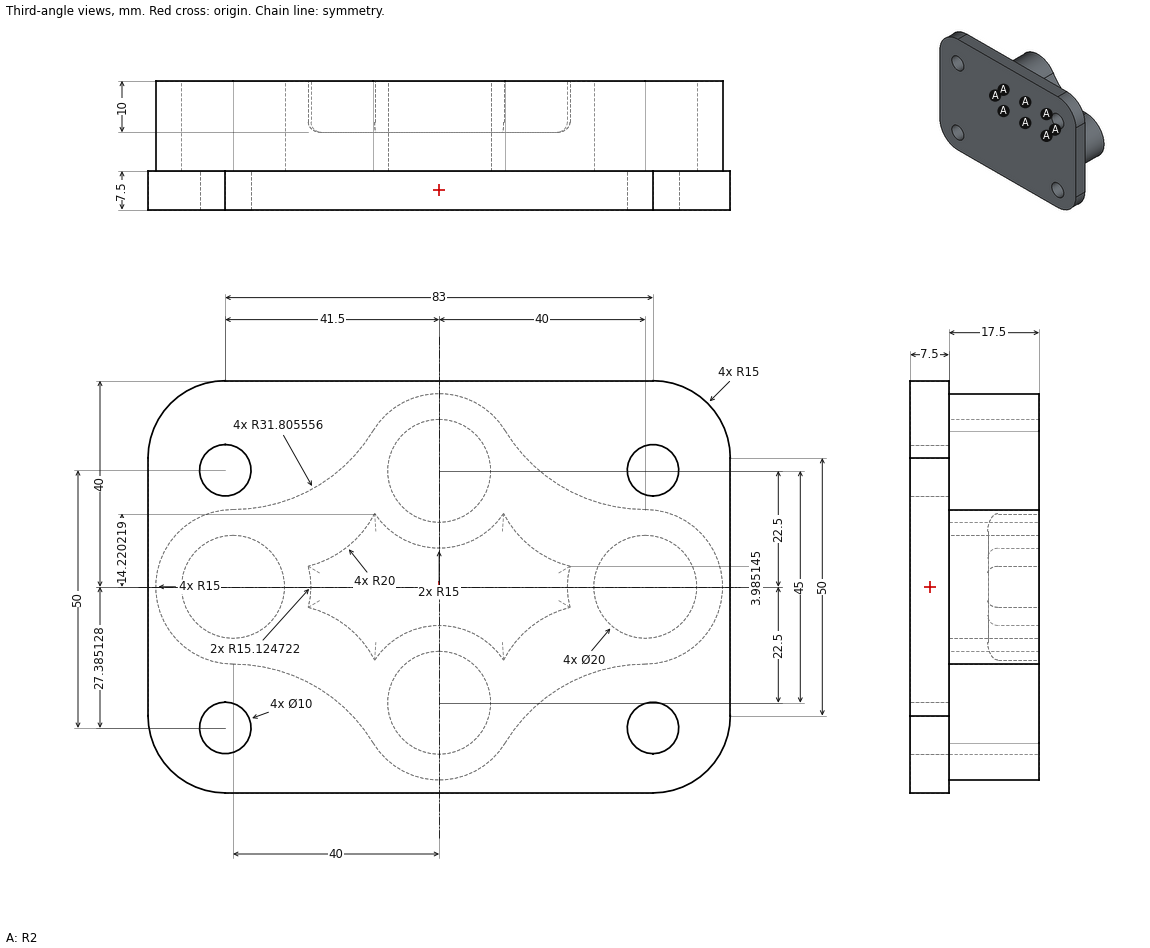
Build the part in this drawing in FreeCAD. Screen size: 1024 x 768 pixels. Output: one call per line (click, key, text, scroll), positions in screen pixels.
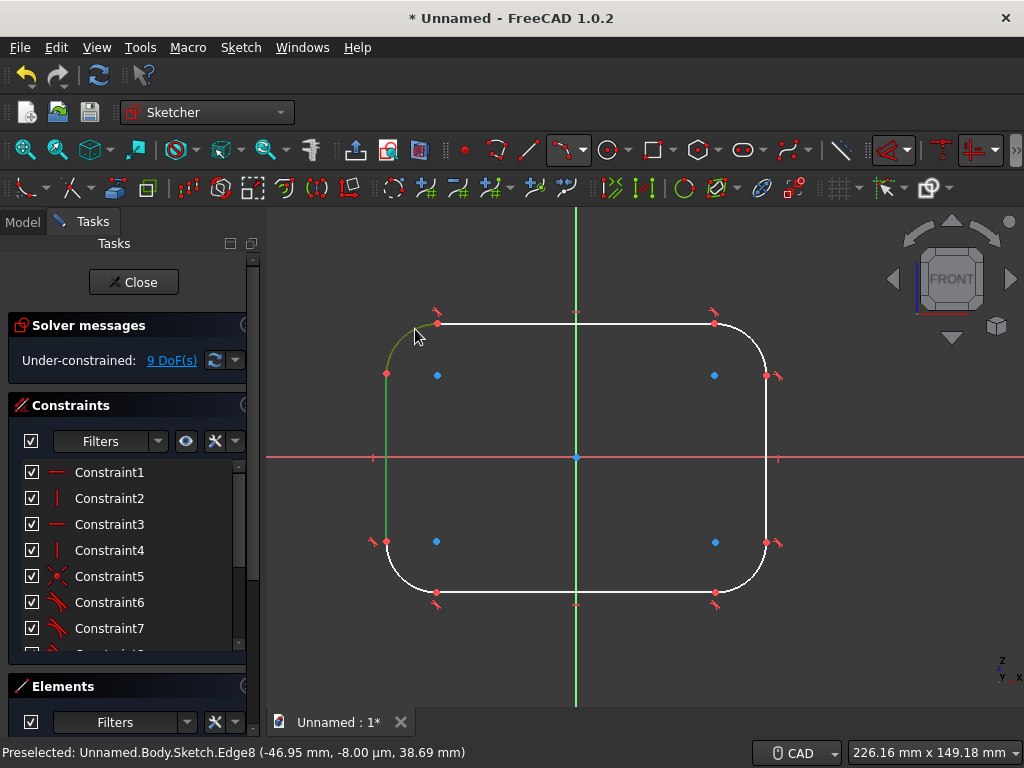
key(t)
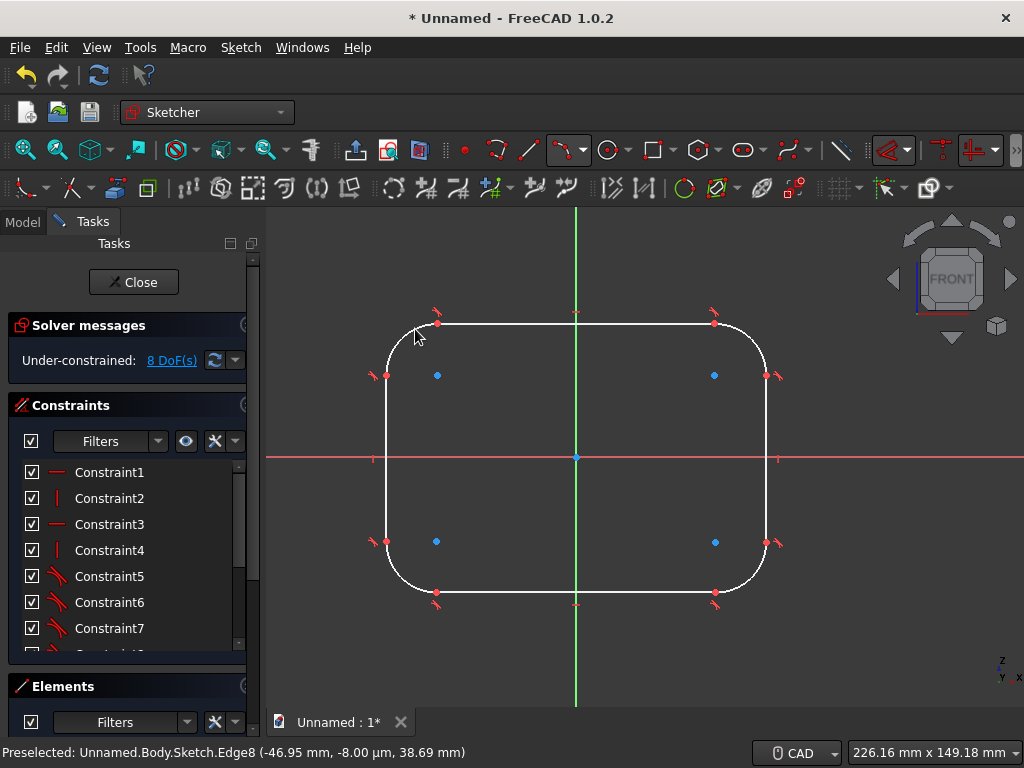
click(761, 352)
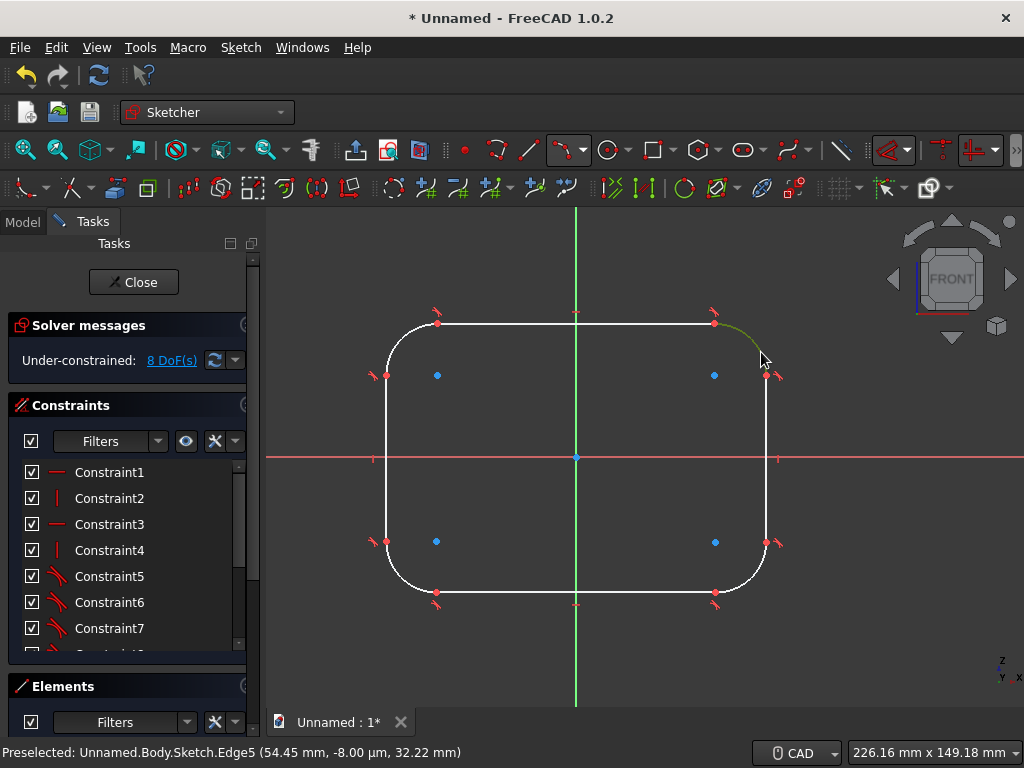
click(739, 587)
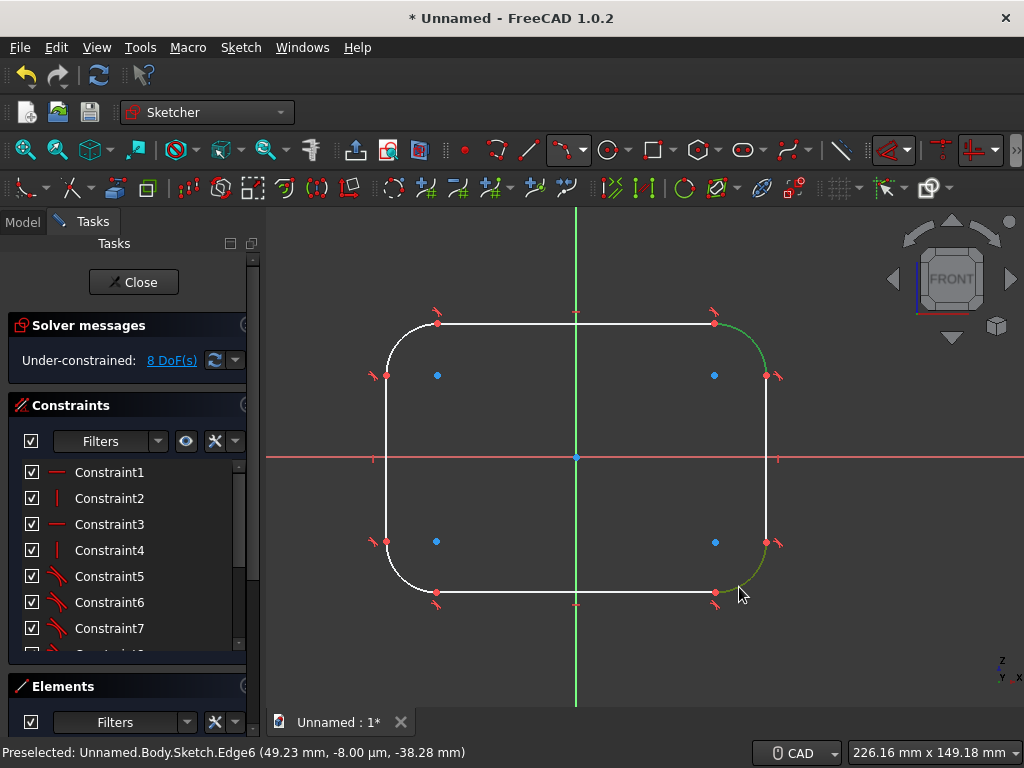
click(392, 565)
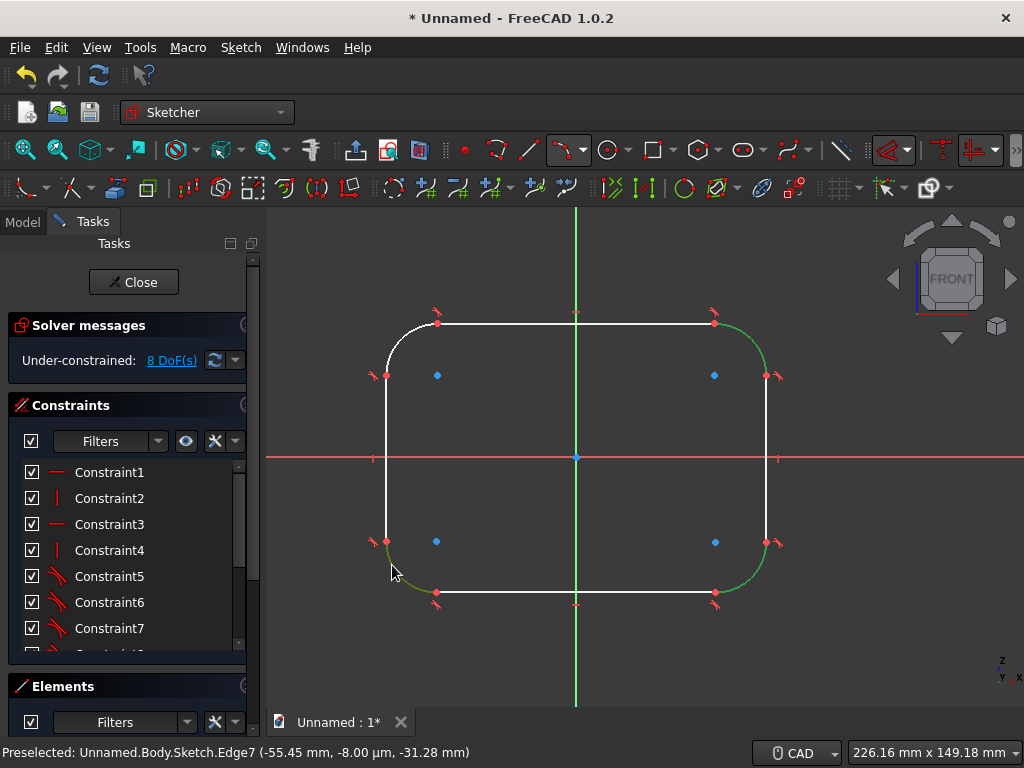
click(414, 330)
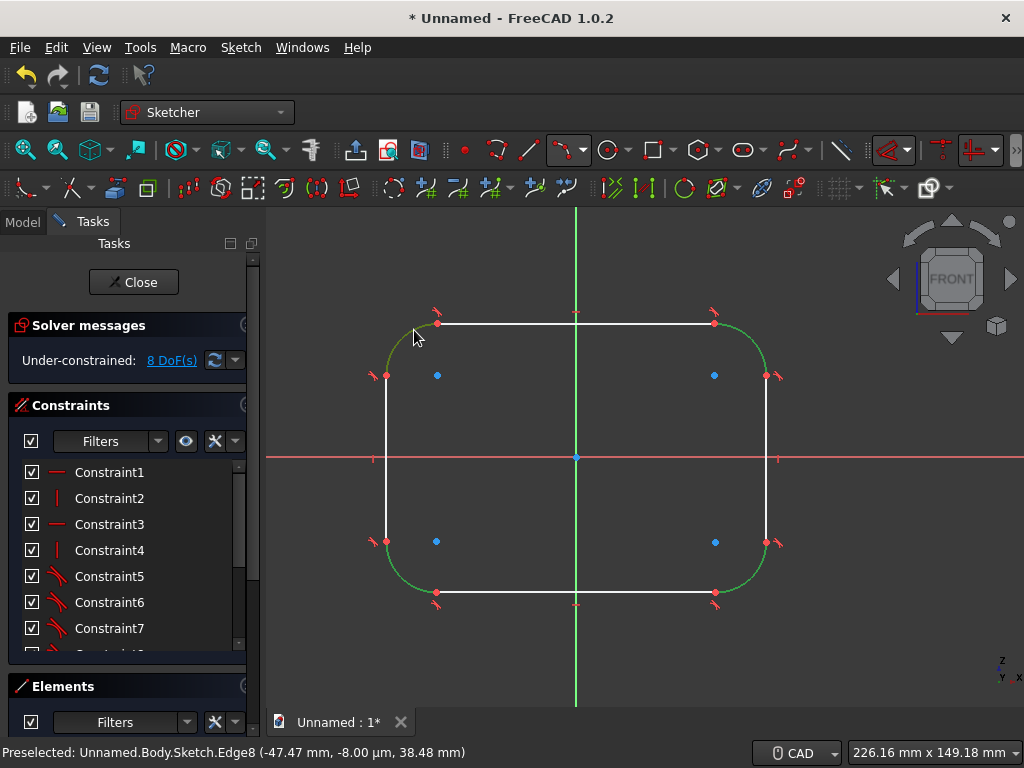
key(e)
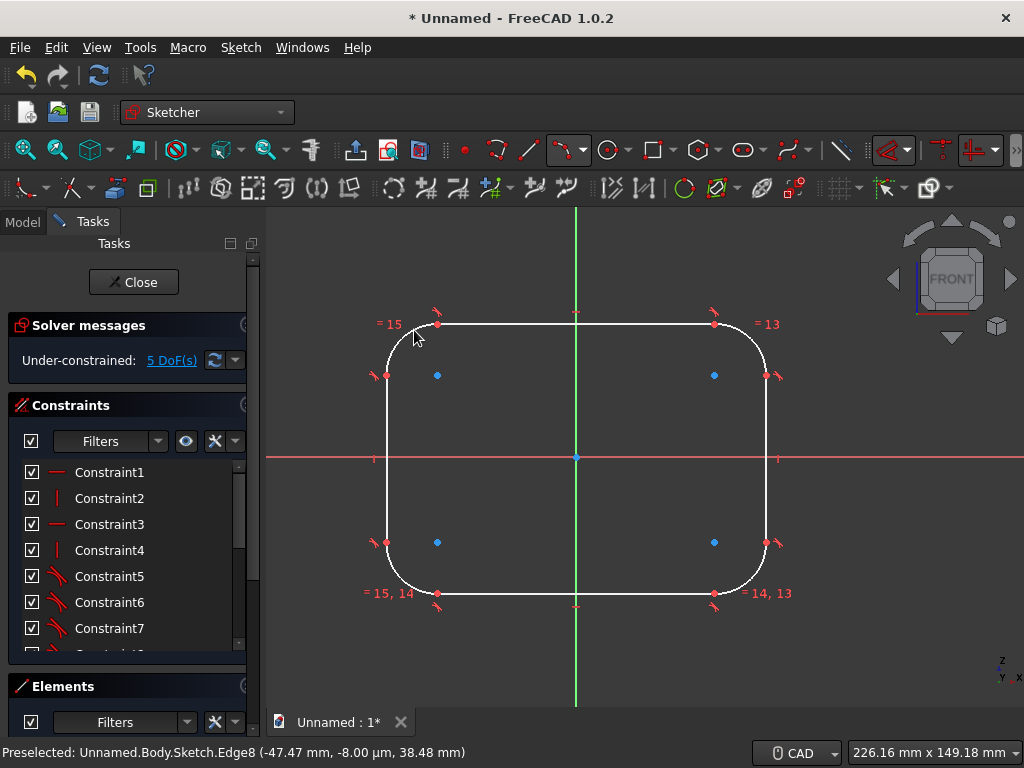
click(760, 352)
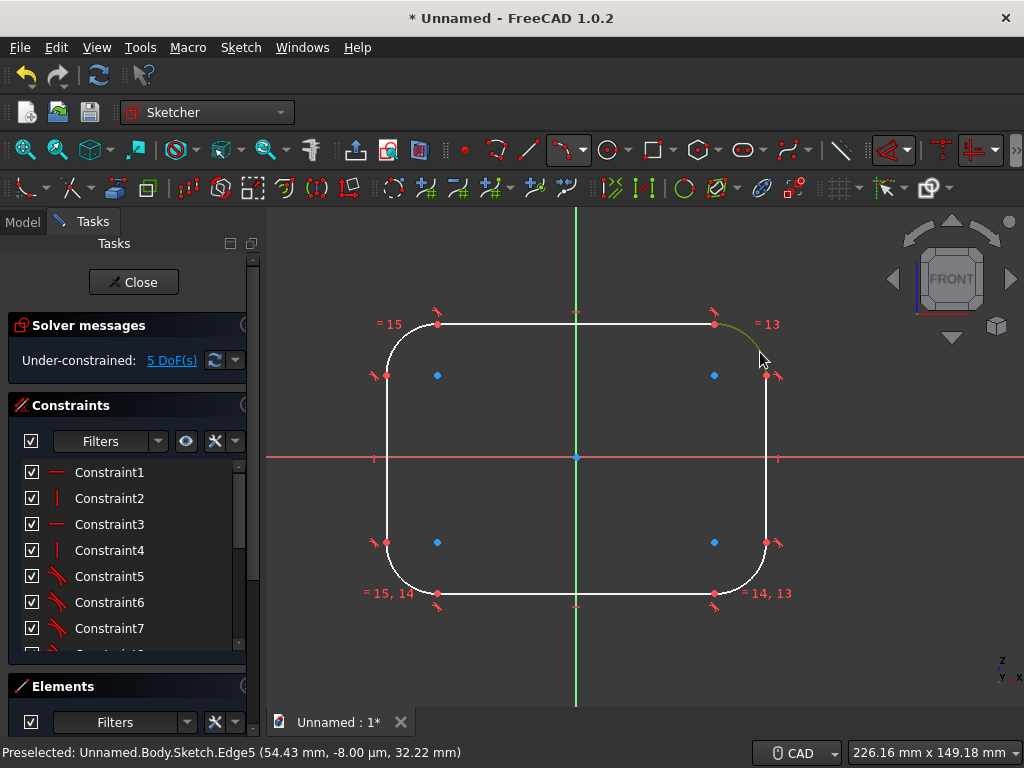
click(910, 150)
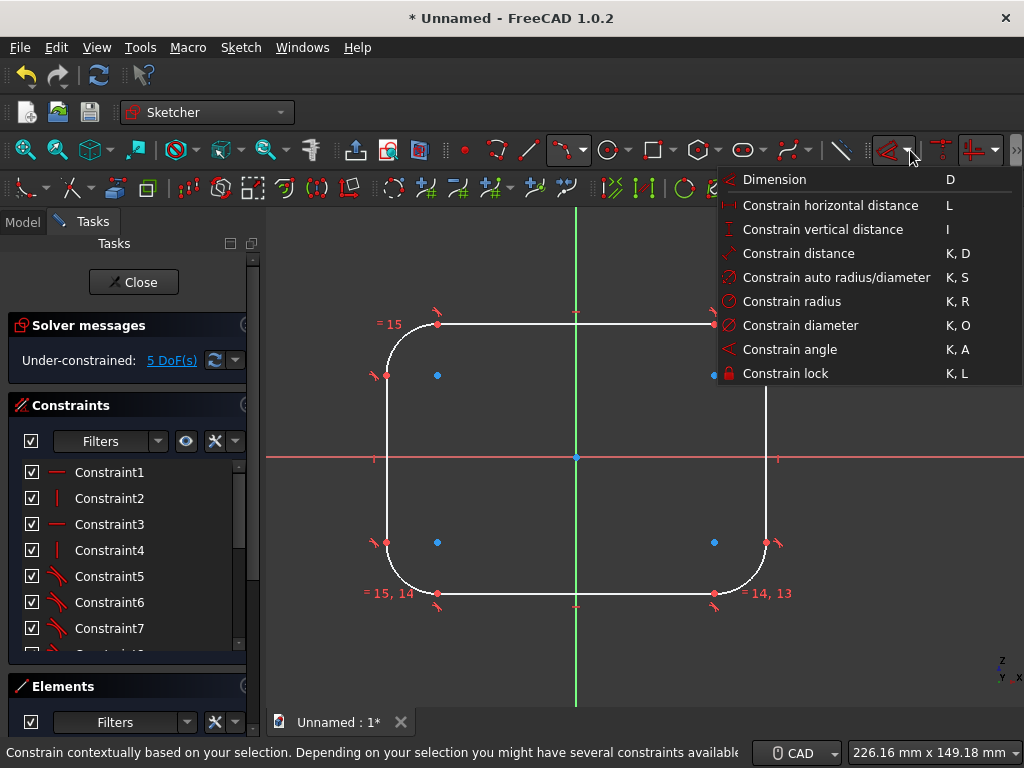
click(870, 301)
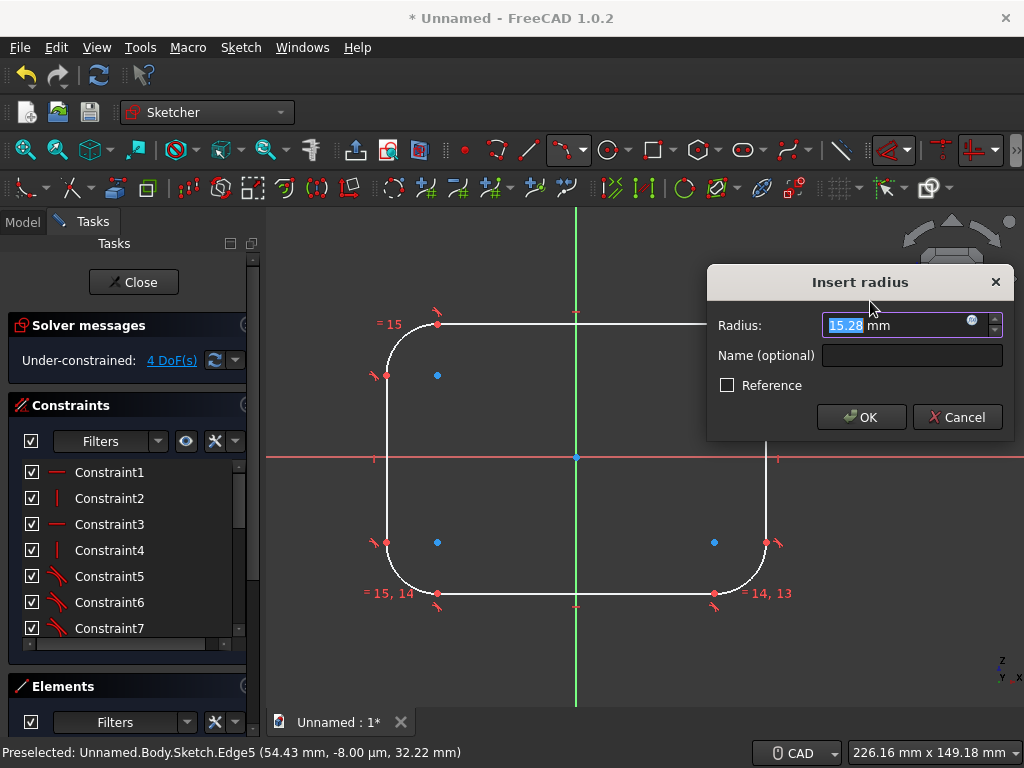
text(15)
key(Return)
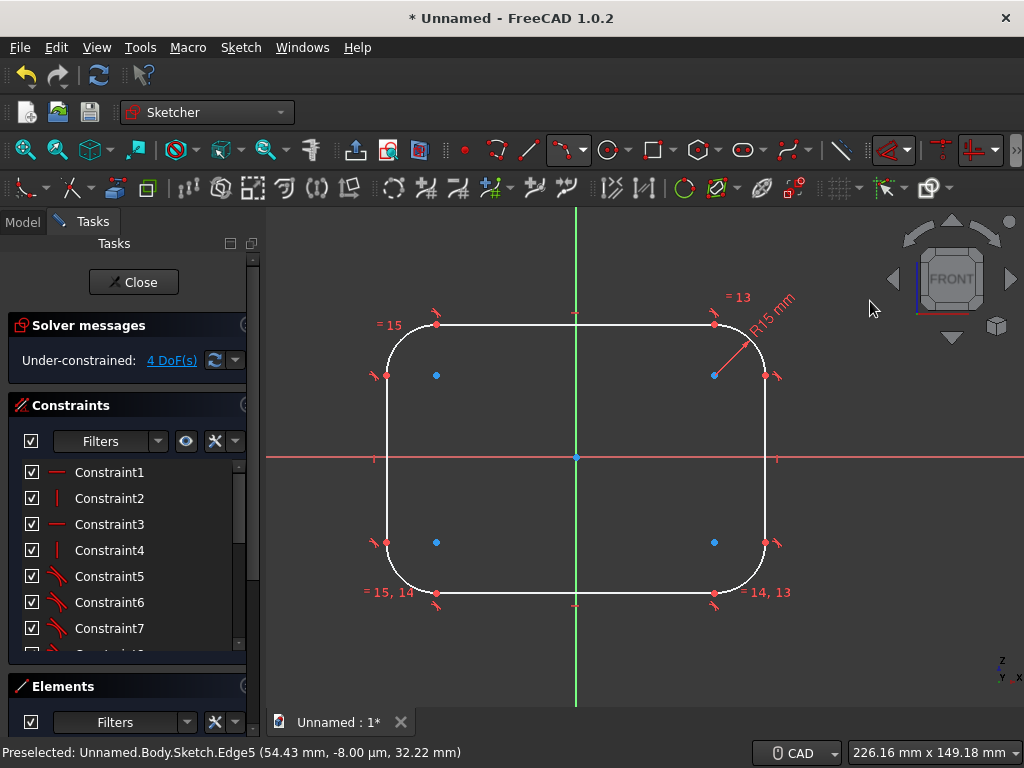
click(520, 325)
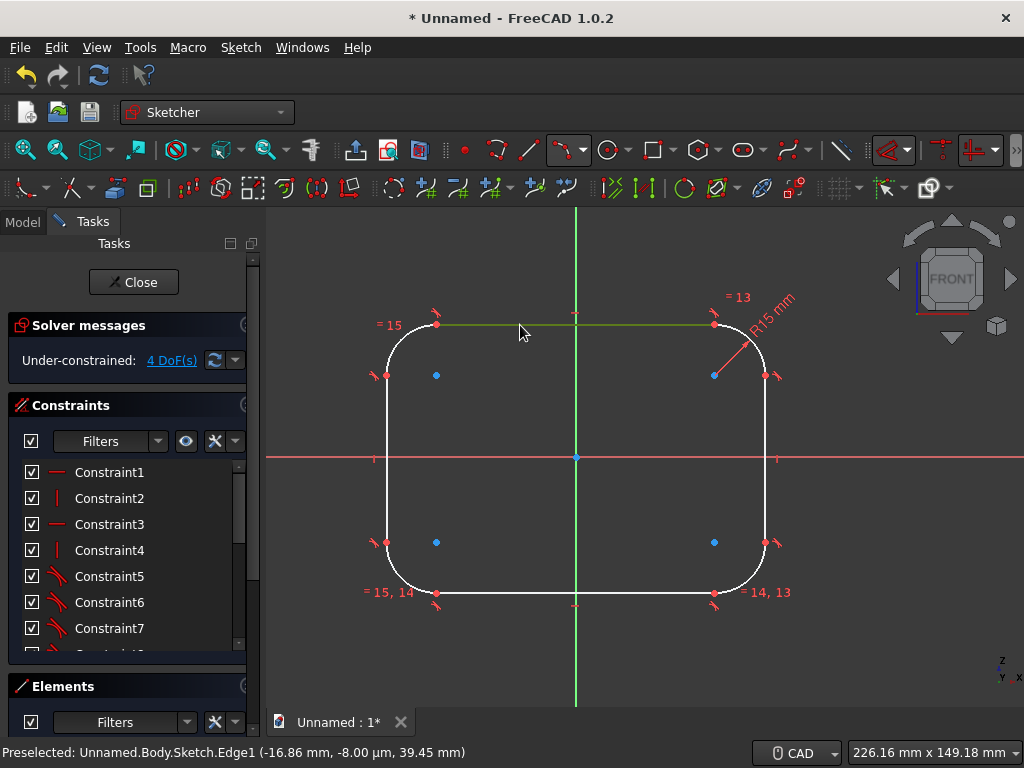
key(l)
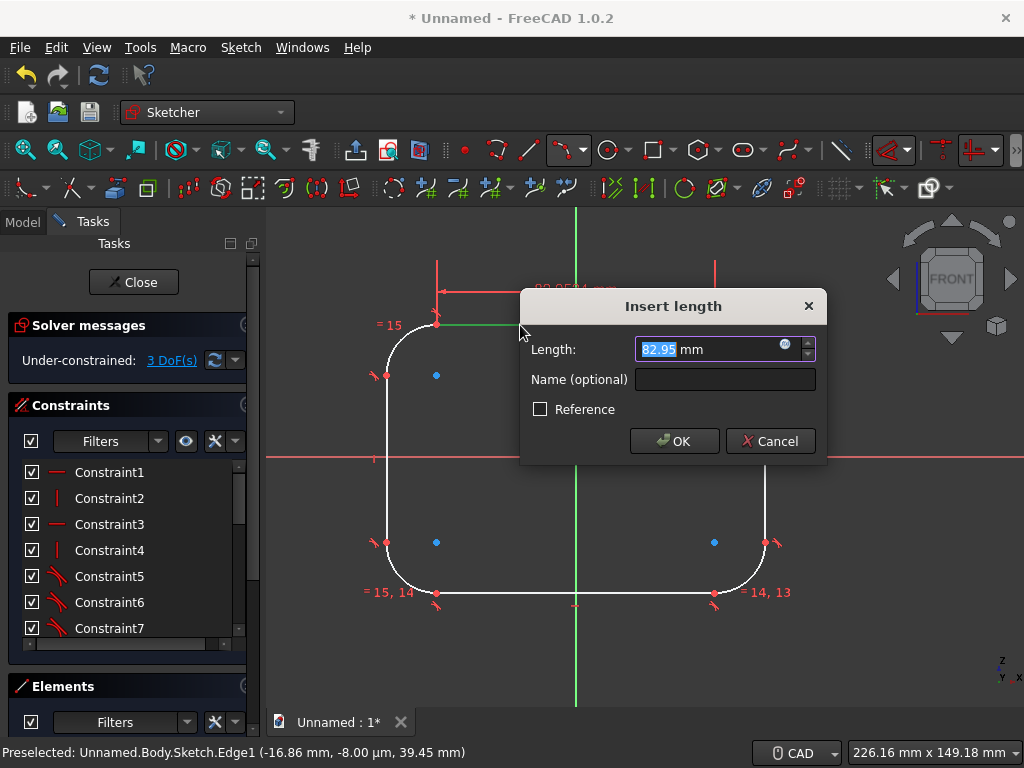
text(83)
key(Return)